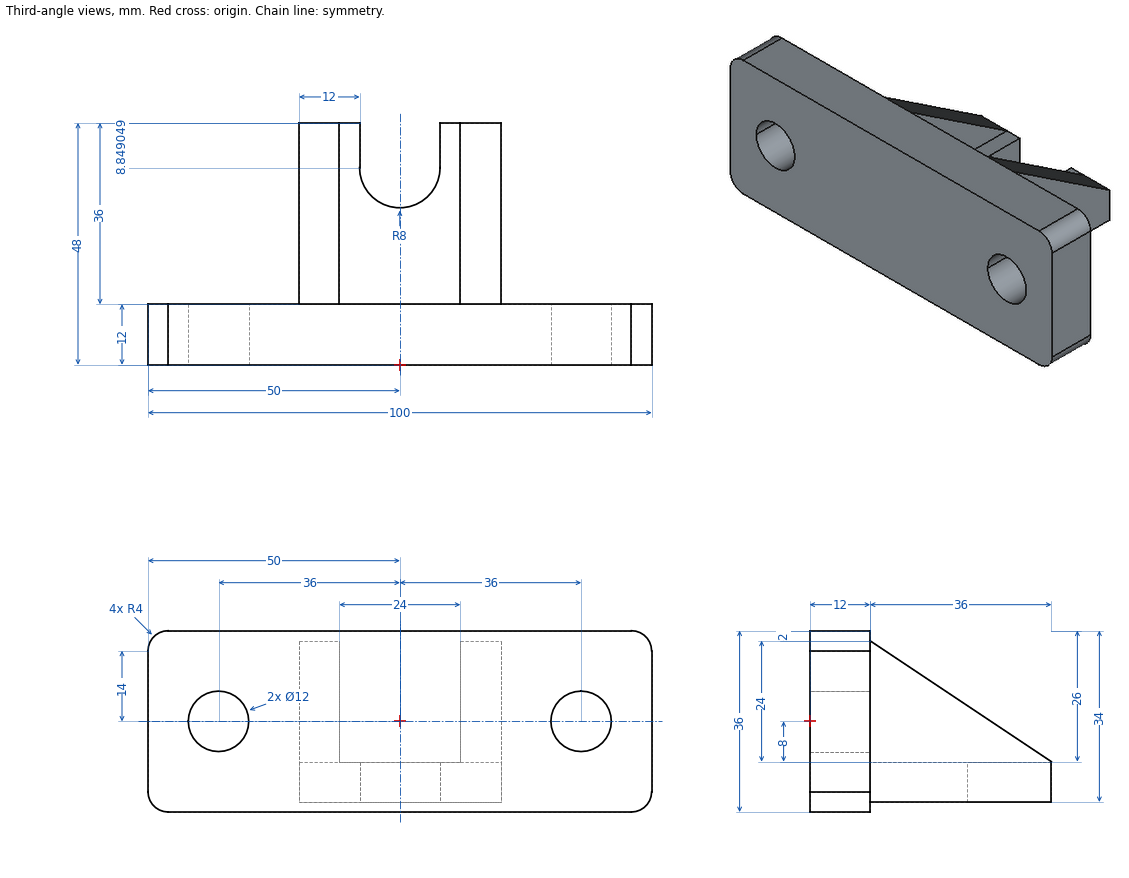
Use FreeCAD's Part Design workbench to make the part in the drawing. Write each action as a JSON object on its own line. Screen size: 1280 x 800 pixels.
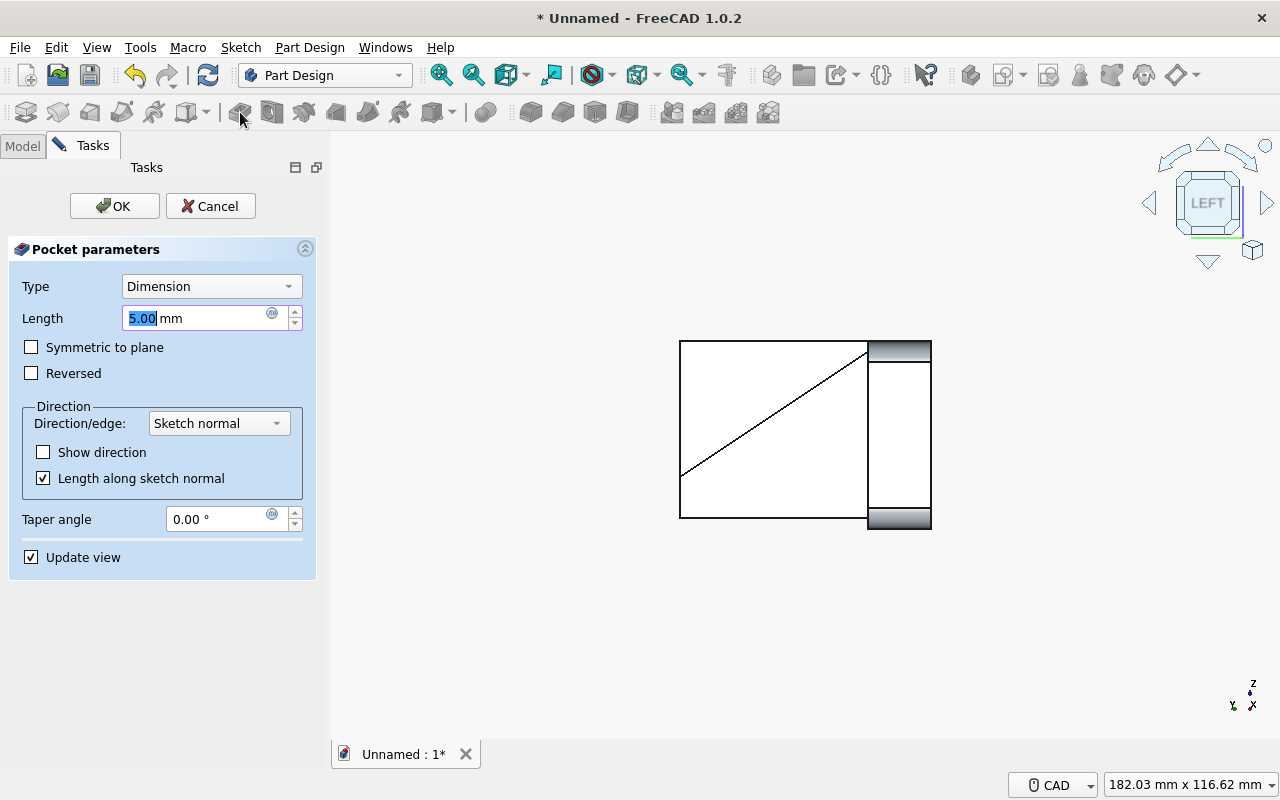
{"action": "left_click", "coordinate": [212, 286]}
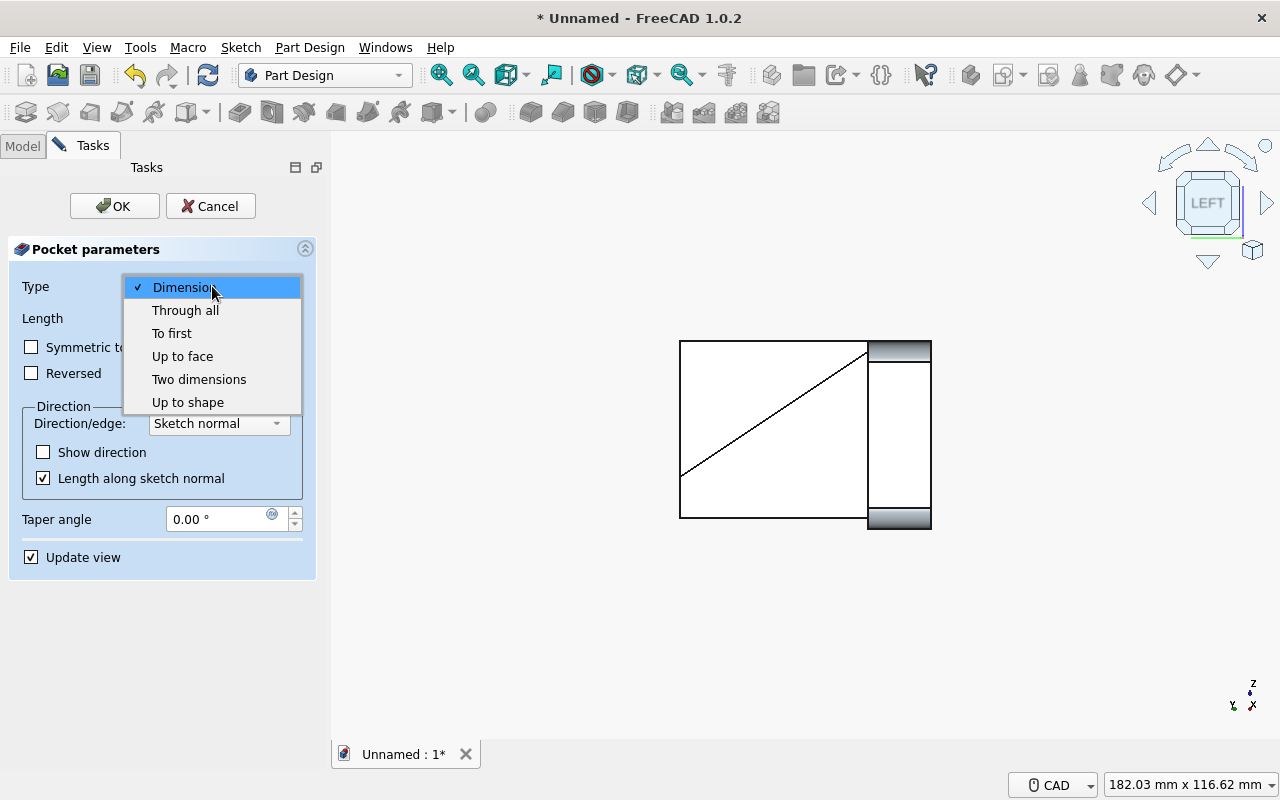
{"action": "left_click", "coordinate": [212, 310]}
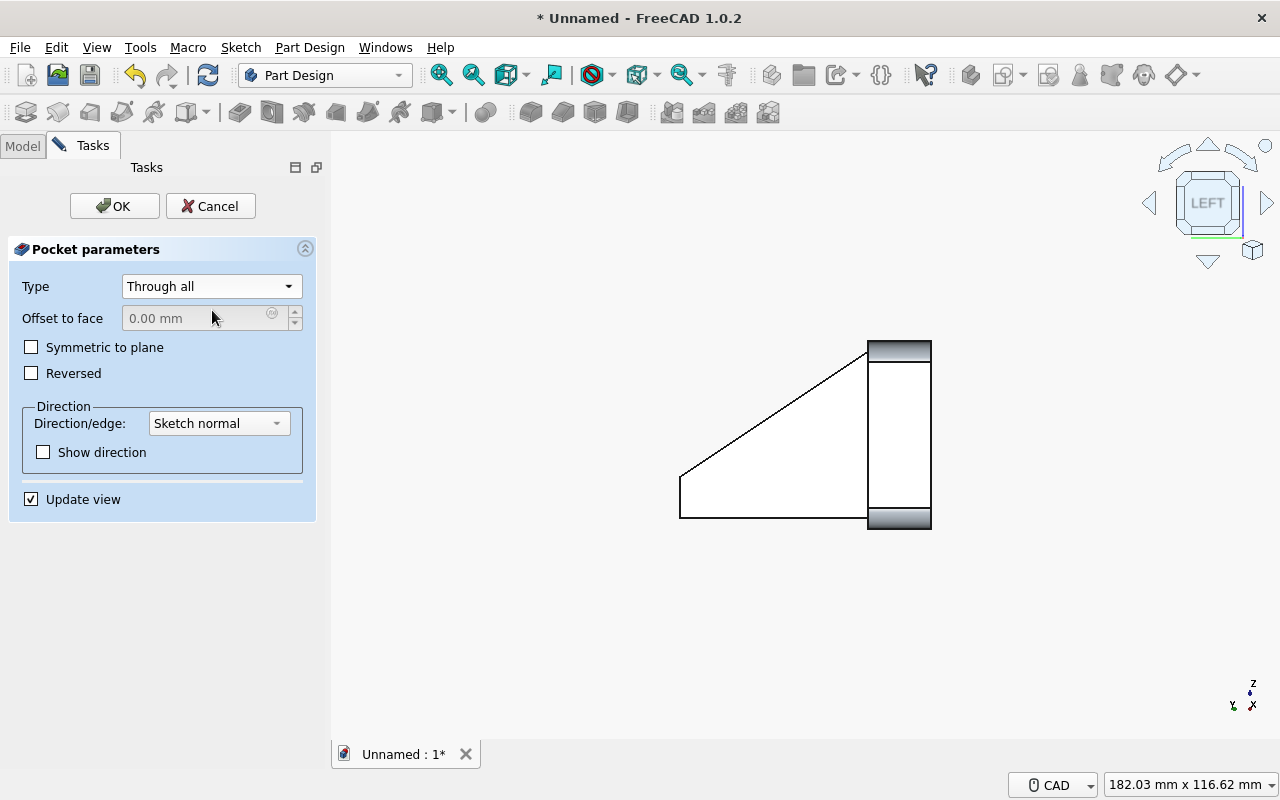
{"action": "left_click", "coordinate": [115, 206]}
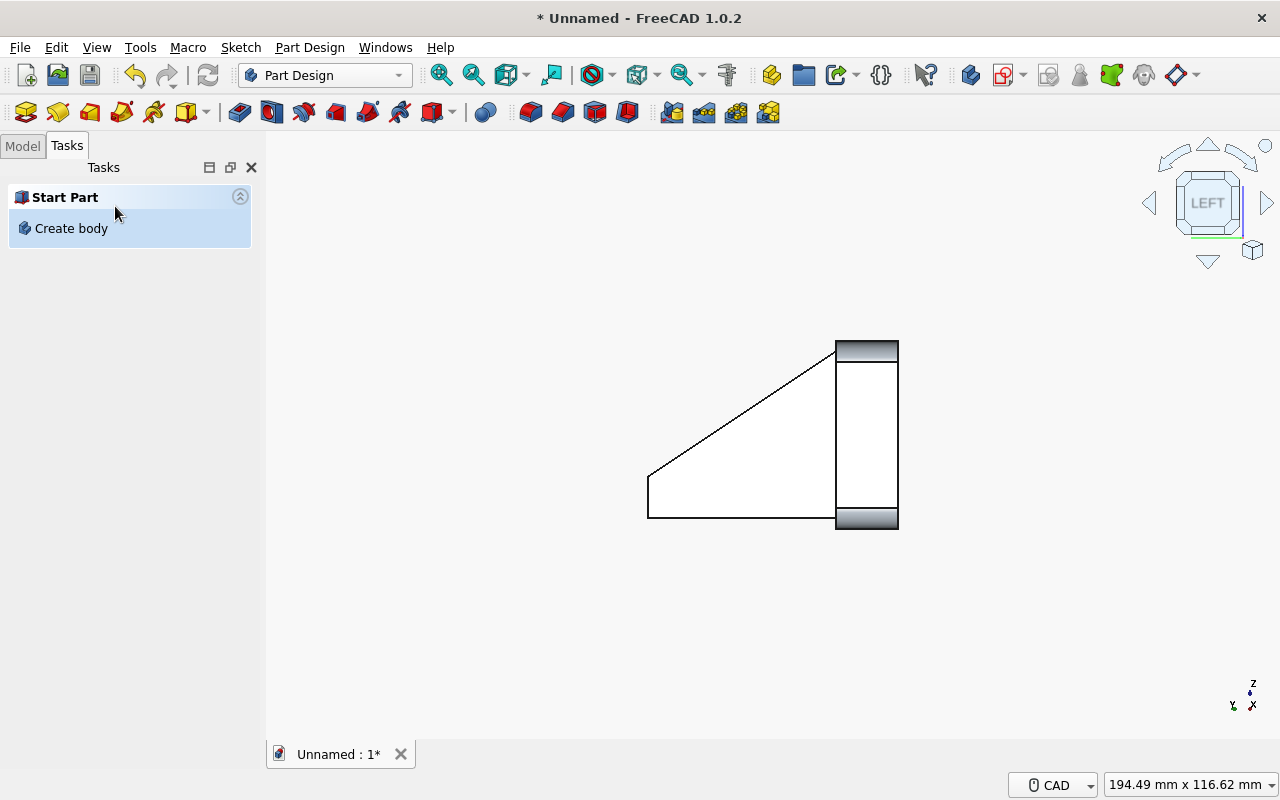
{"action": "left_click", "coordinate": [442, 76]}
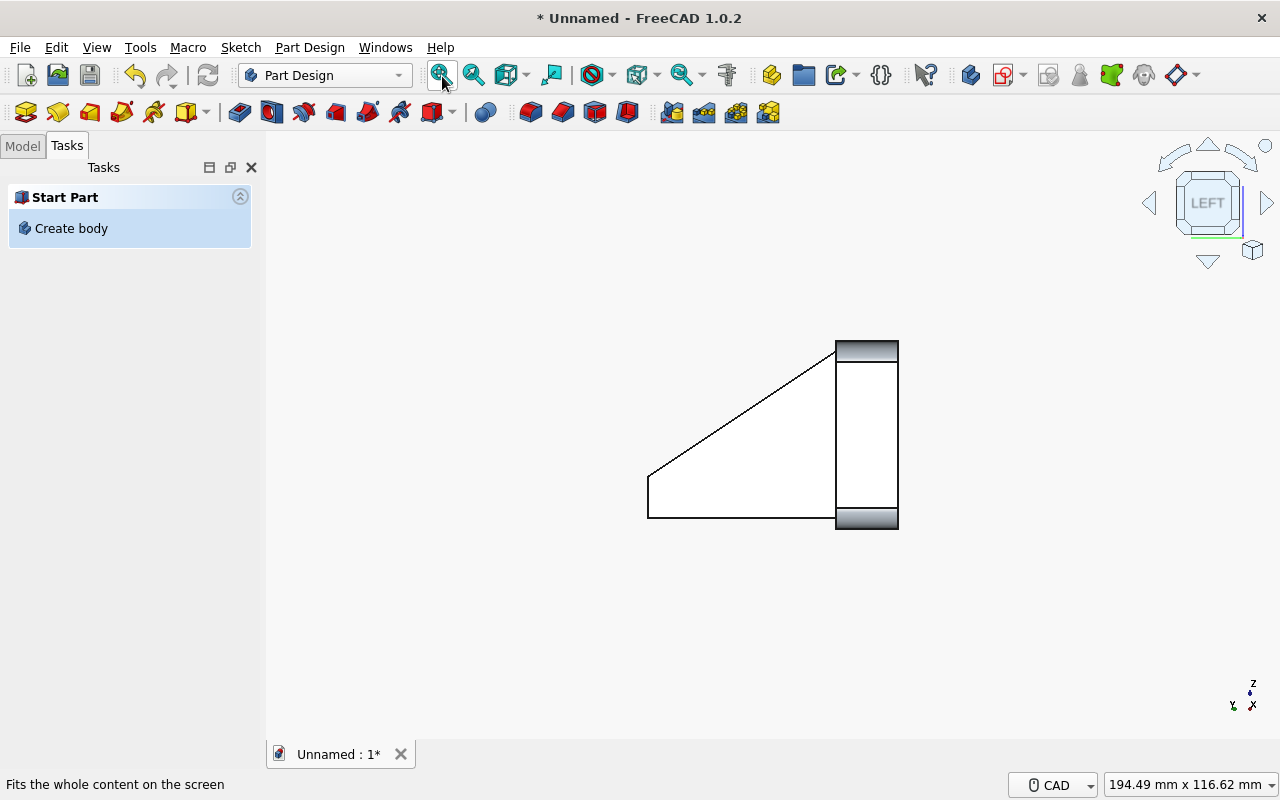
{"action": "left_click", "coordinate": [1004, 76]}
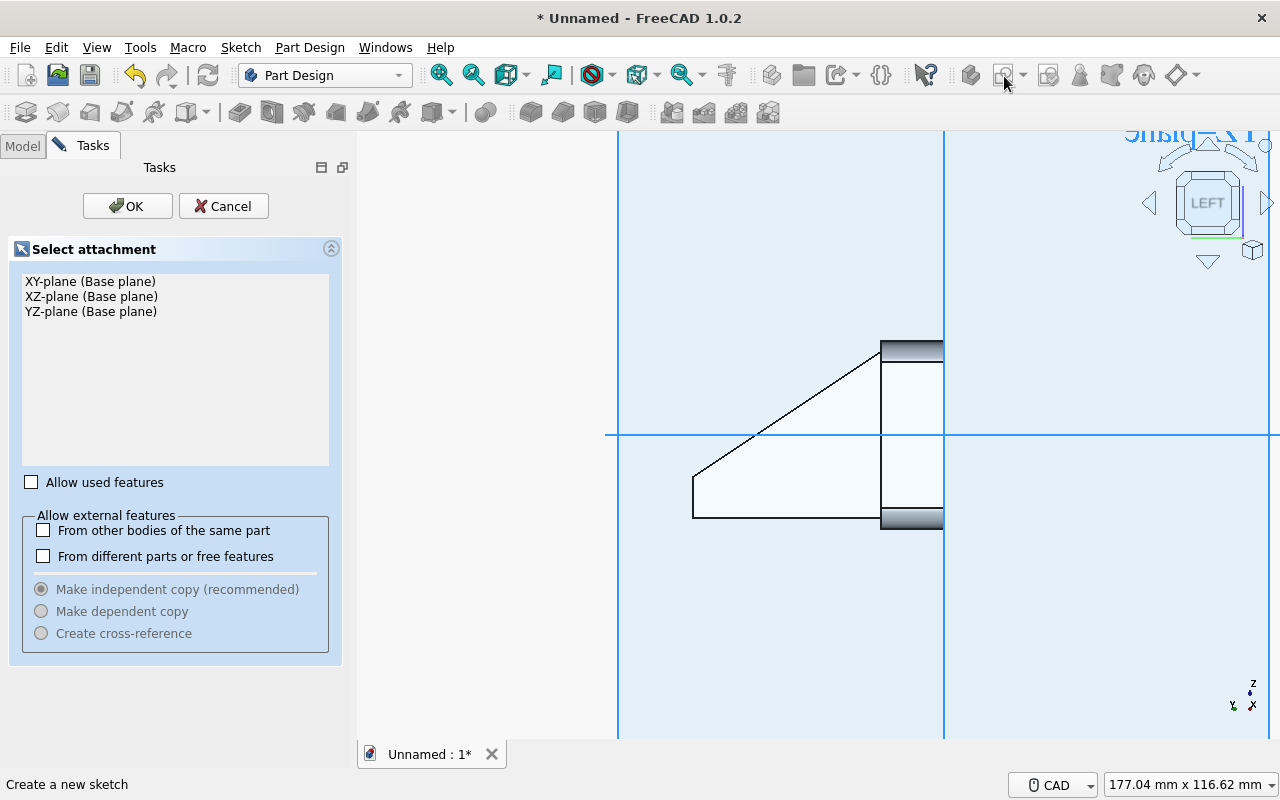
{"action": "left_click", "coordinate": [82, 312]}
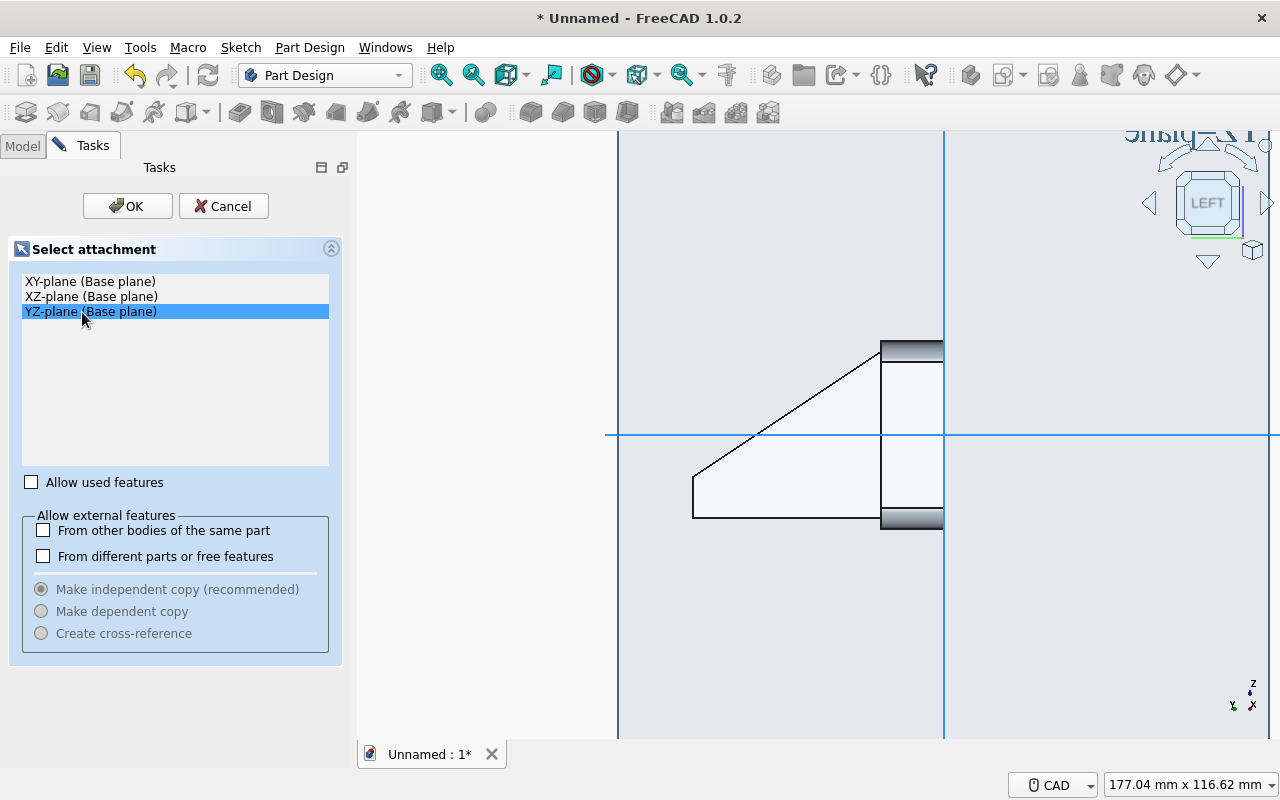
{"action": "left_click", "coordinate": [128, 206]}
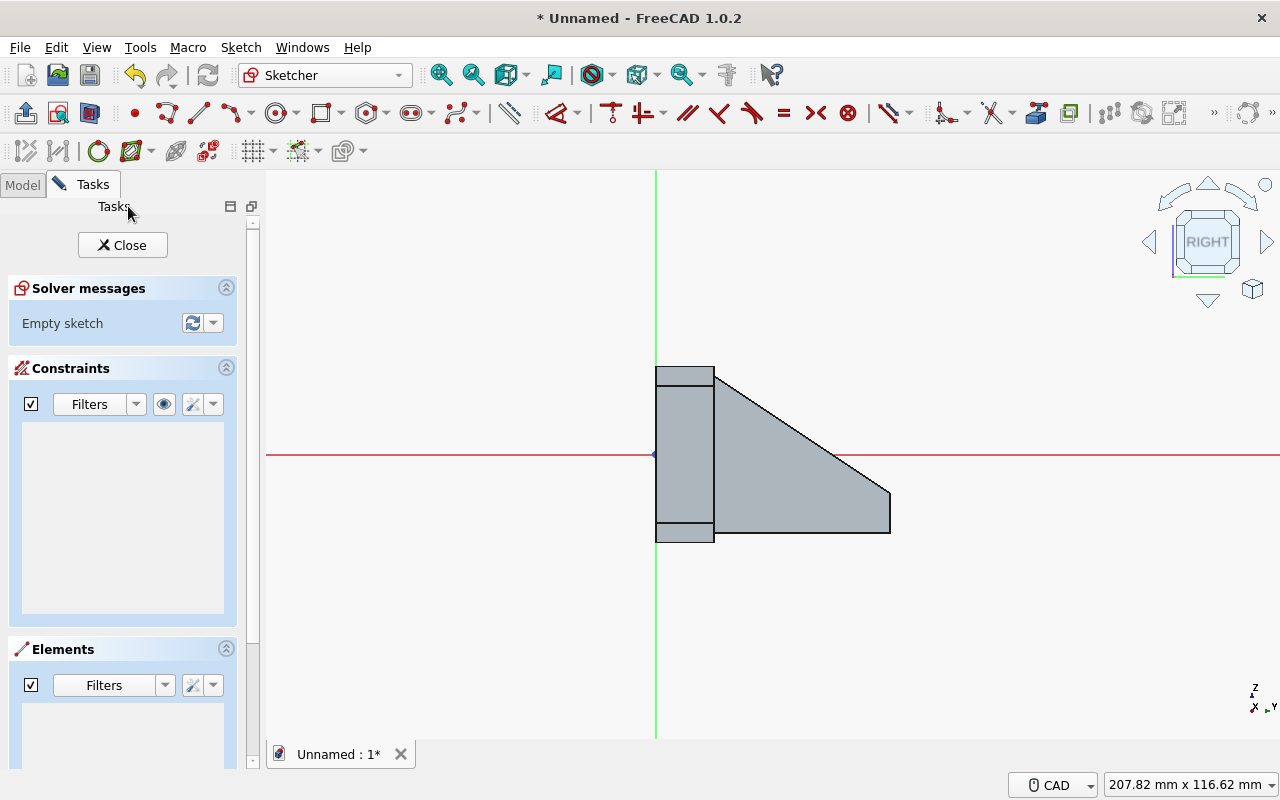
{"action": "left_click", "coordinate": [90, 114]}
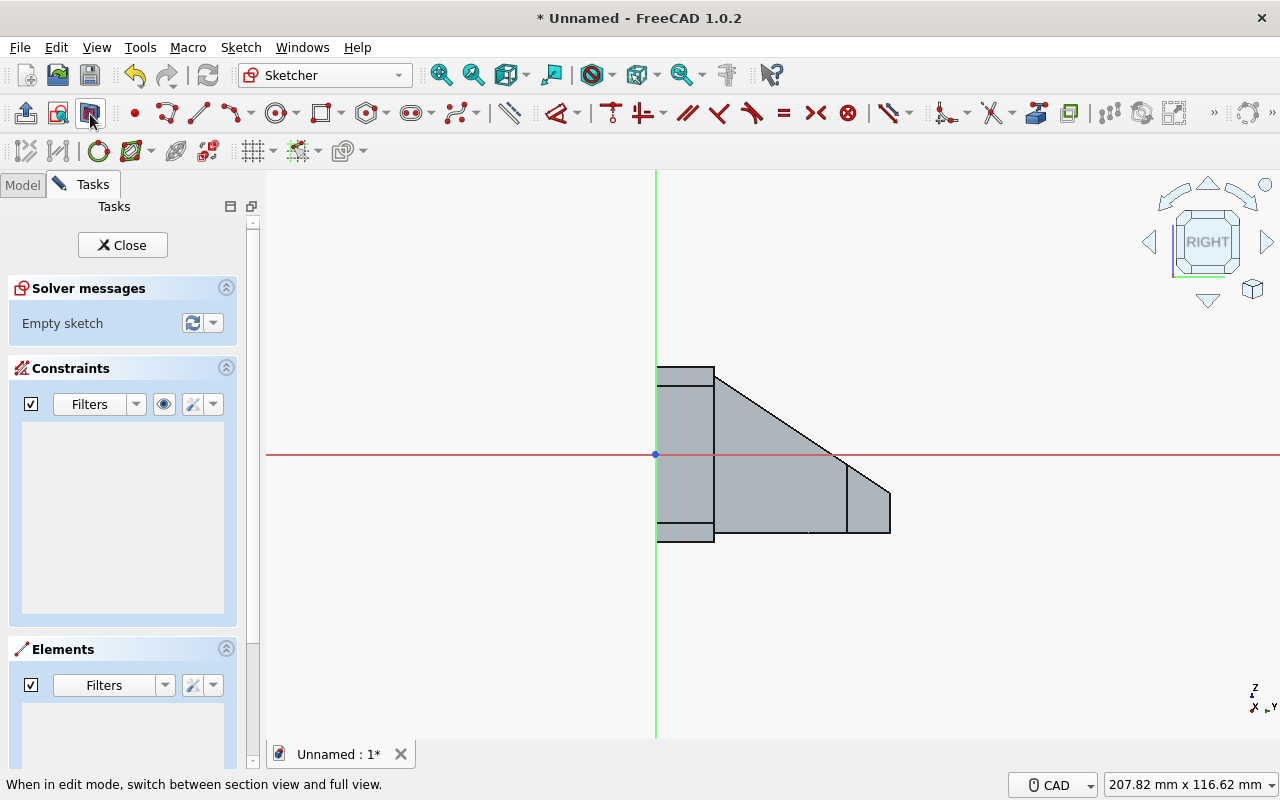
{"action": "scroll", "coordinate": [813, 424], "scroll_direction": "up", "scroll_amount": 5}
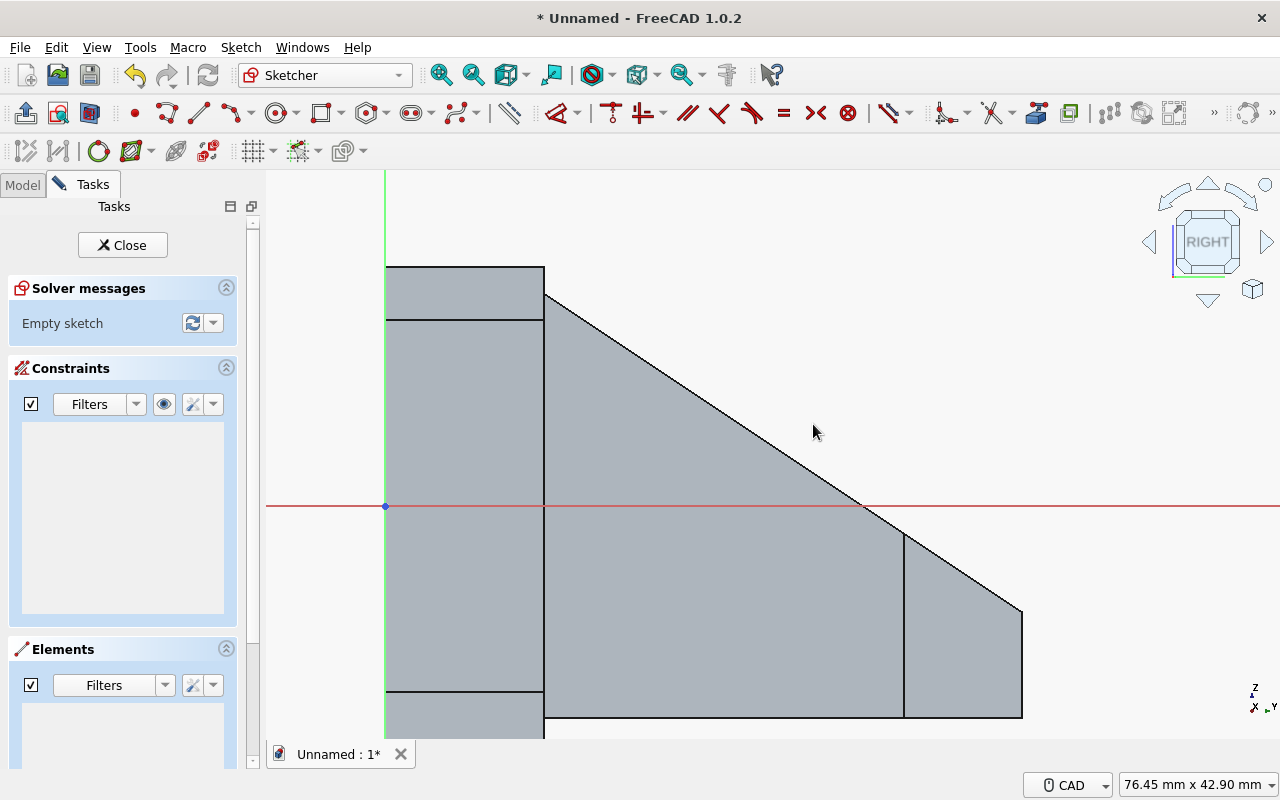
{"action": "left_click", "coordinate": [168, 114]}